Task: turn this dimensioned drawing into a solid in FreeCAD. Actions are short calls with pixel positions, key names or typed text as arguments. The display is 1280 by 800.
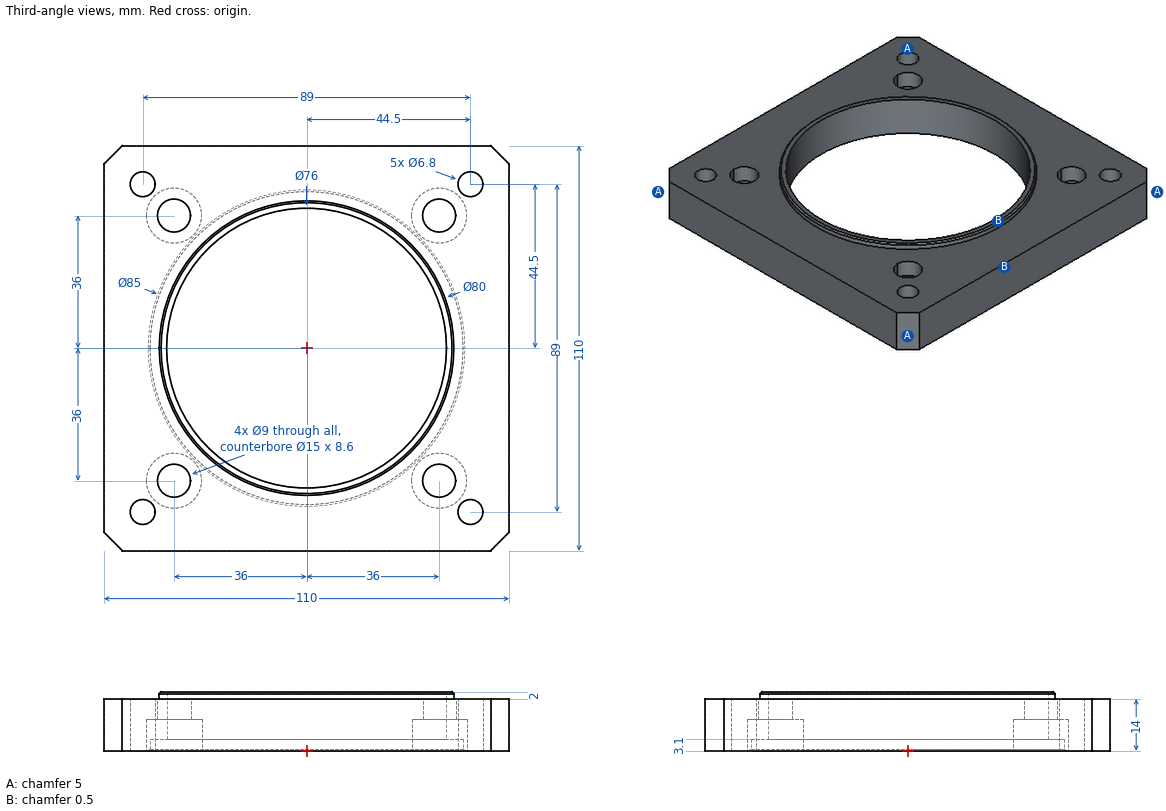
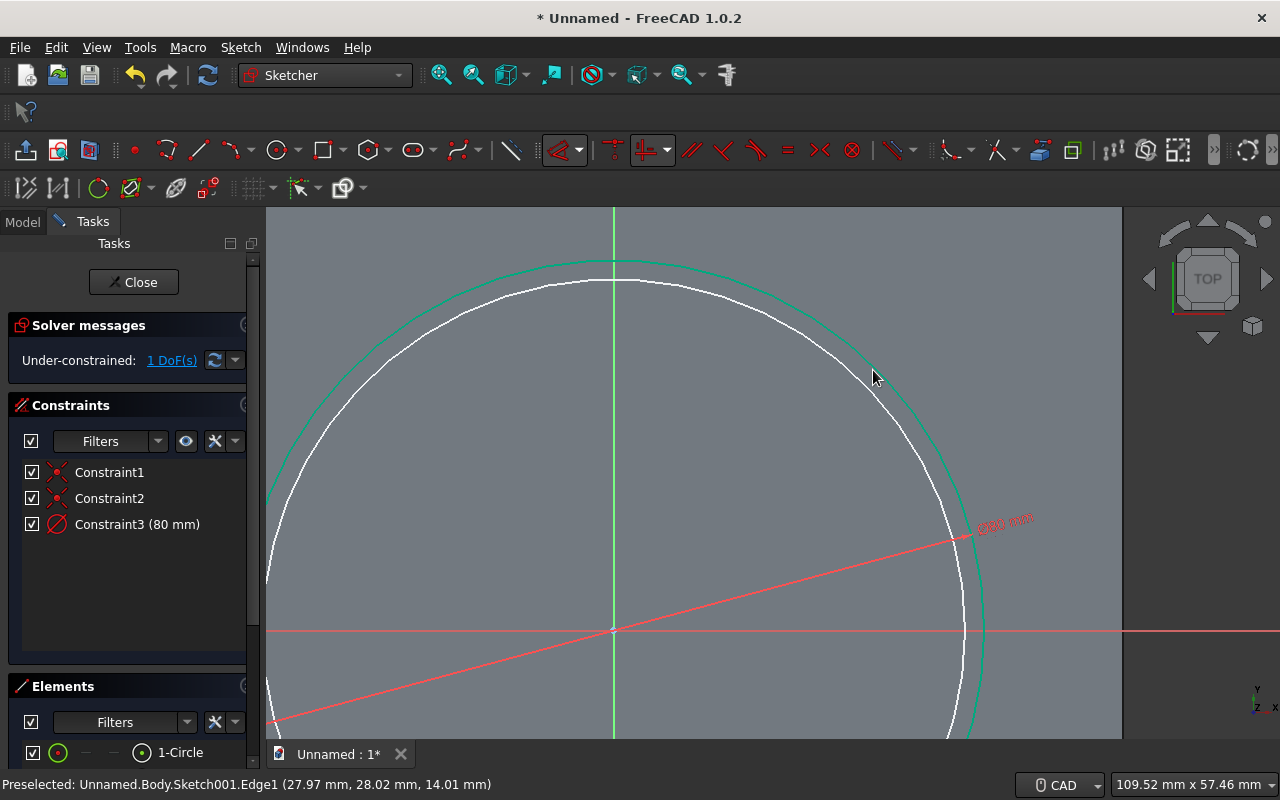
click(861, 381)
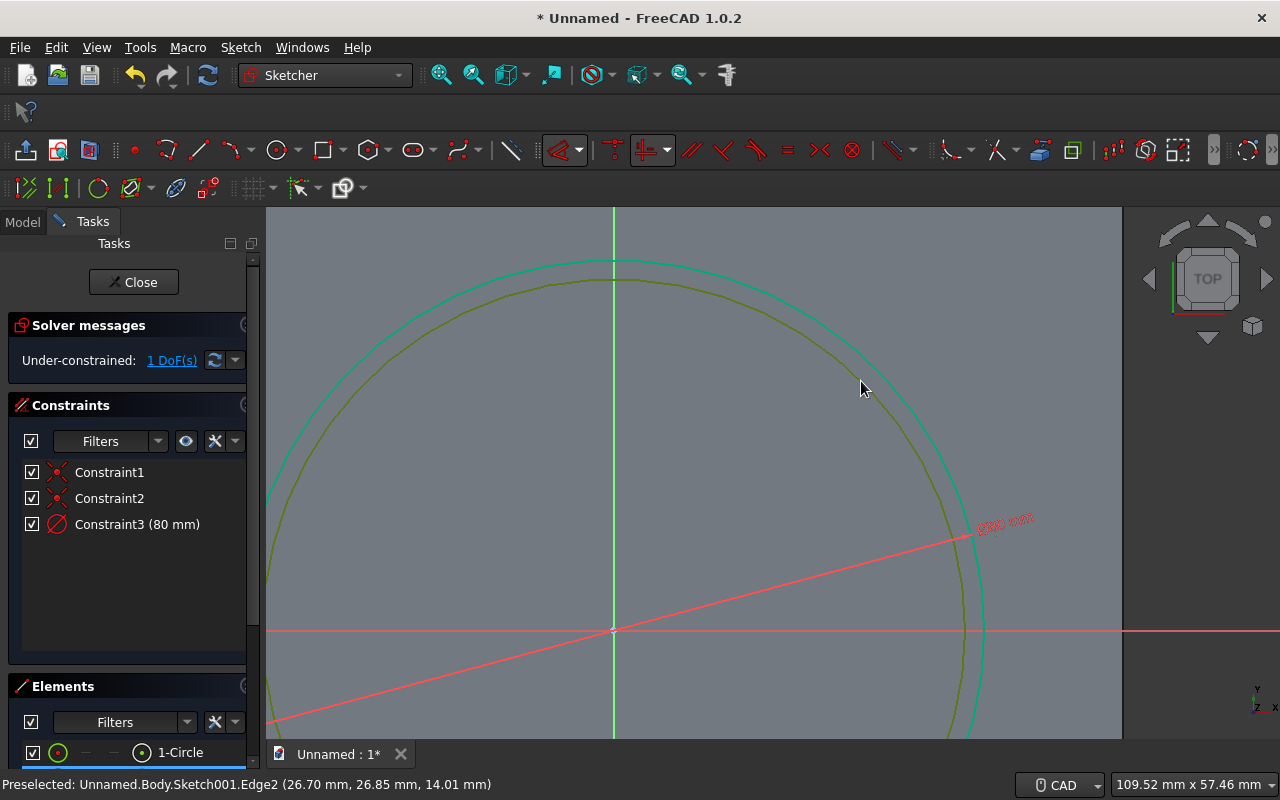
click(582, 150)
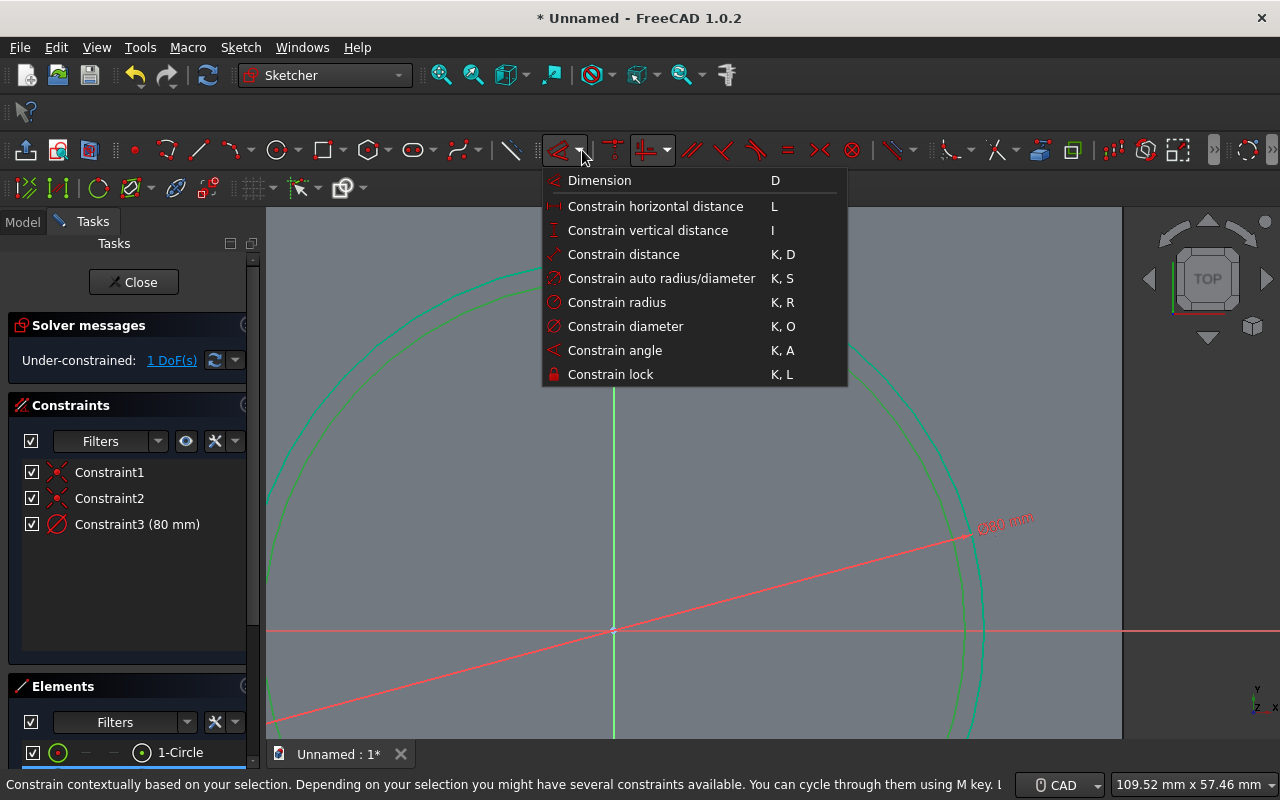
click(695, 326)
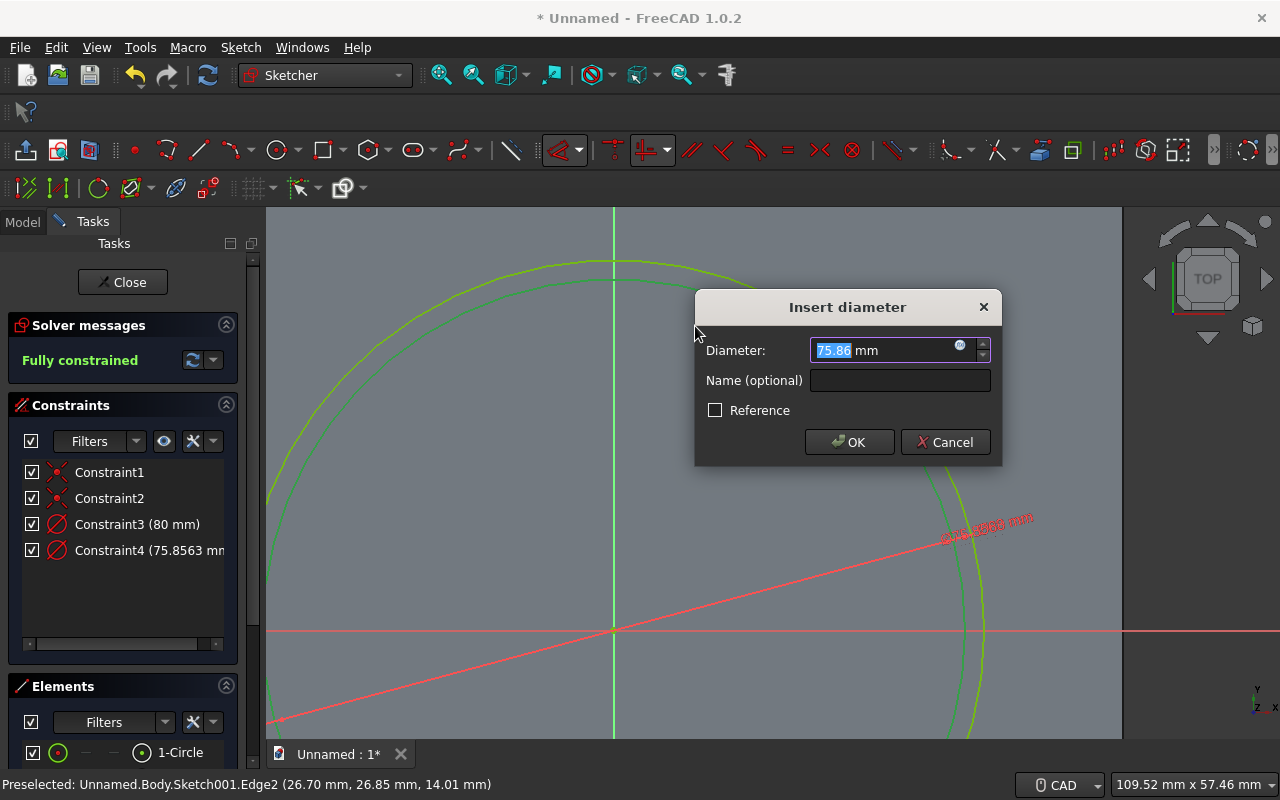
text(76)
key(Return)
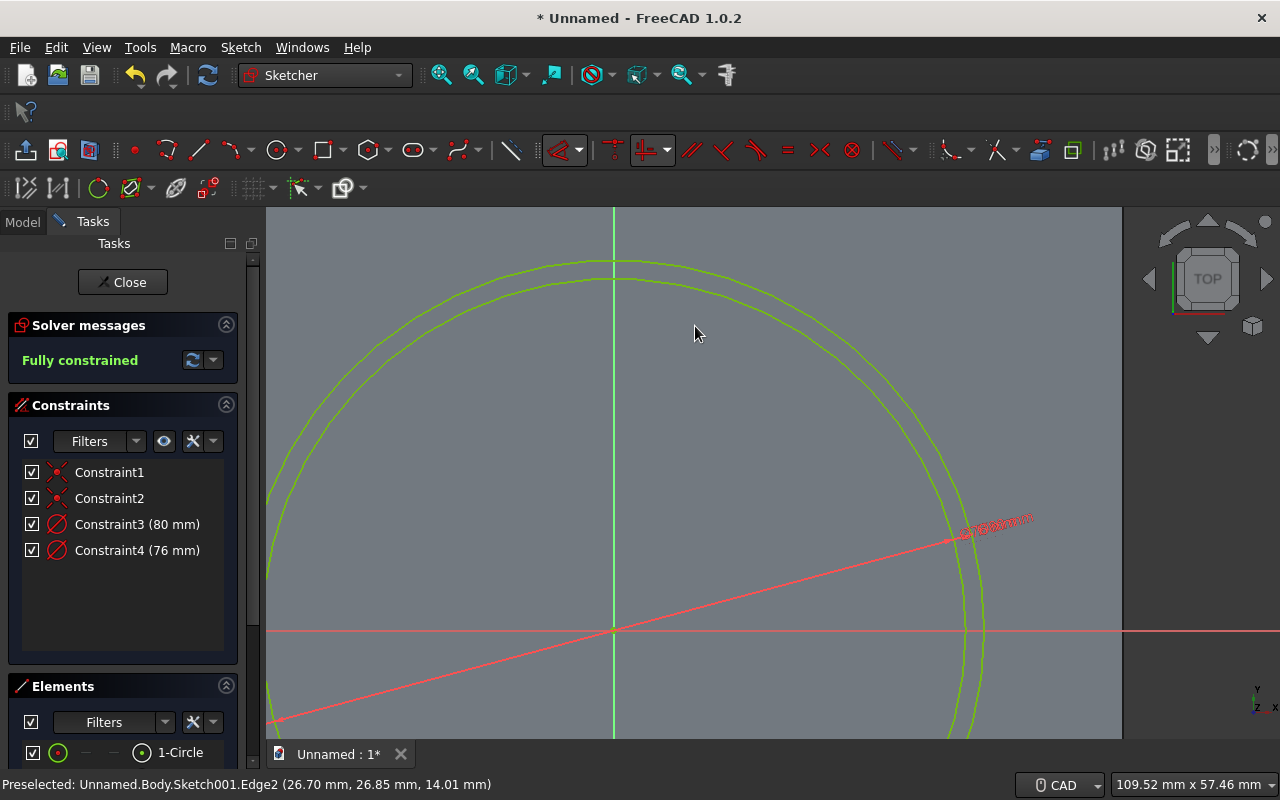
click(123, 282)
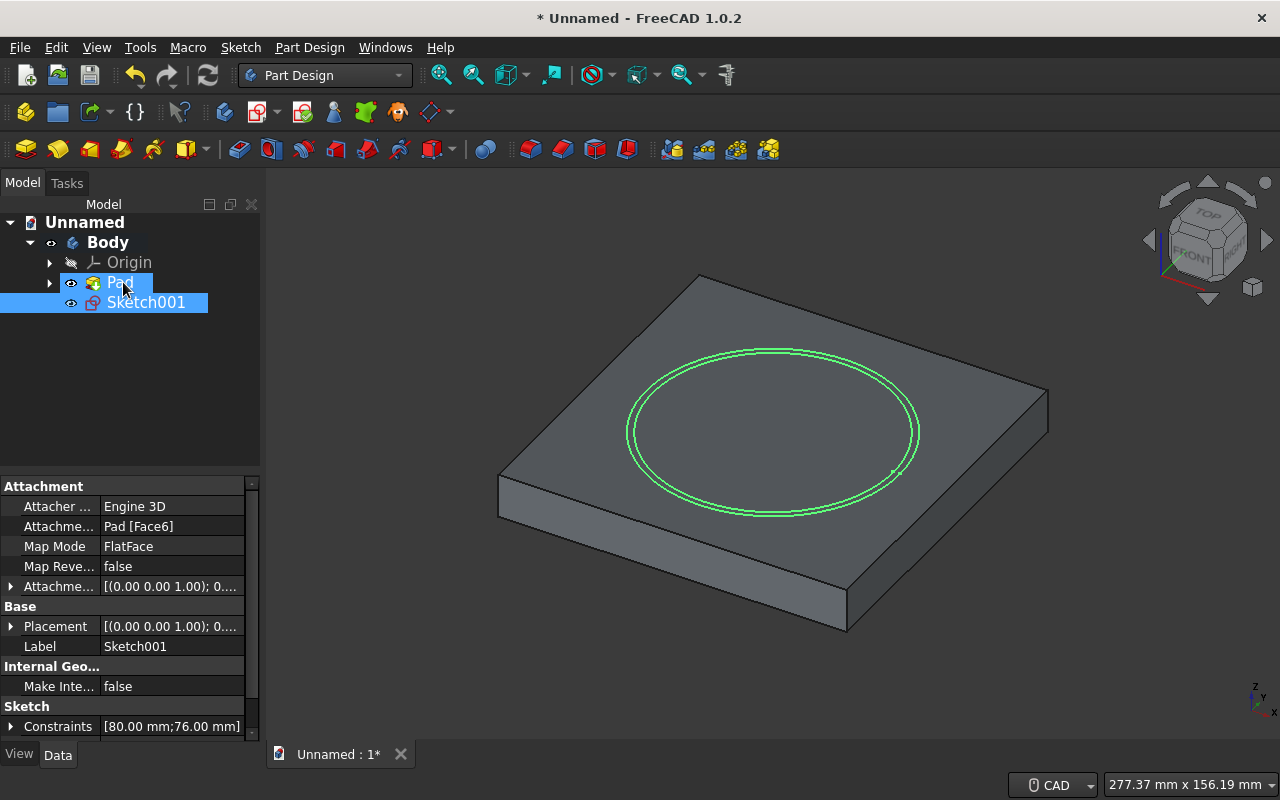
click(26, 150)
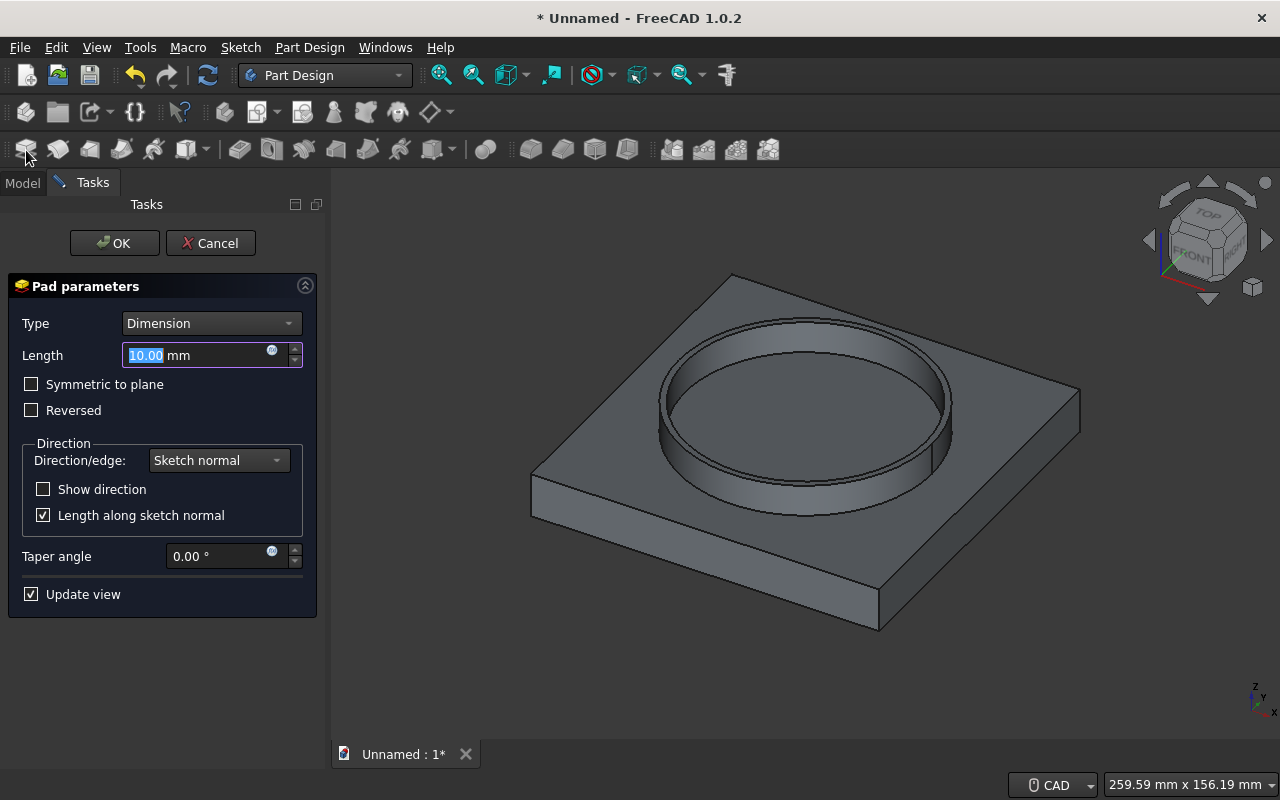
text(2)
key(Tab)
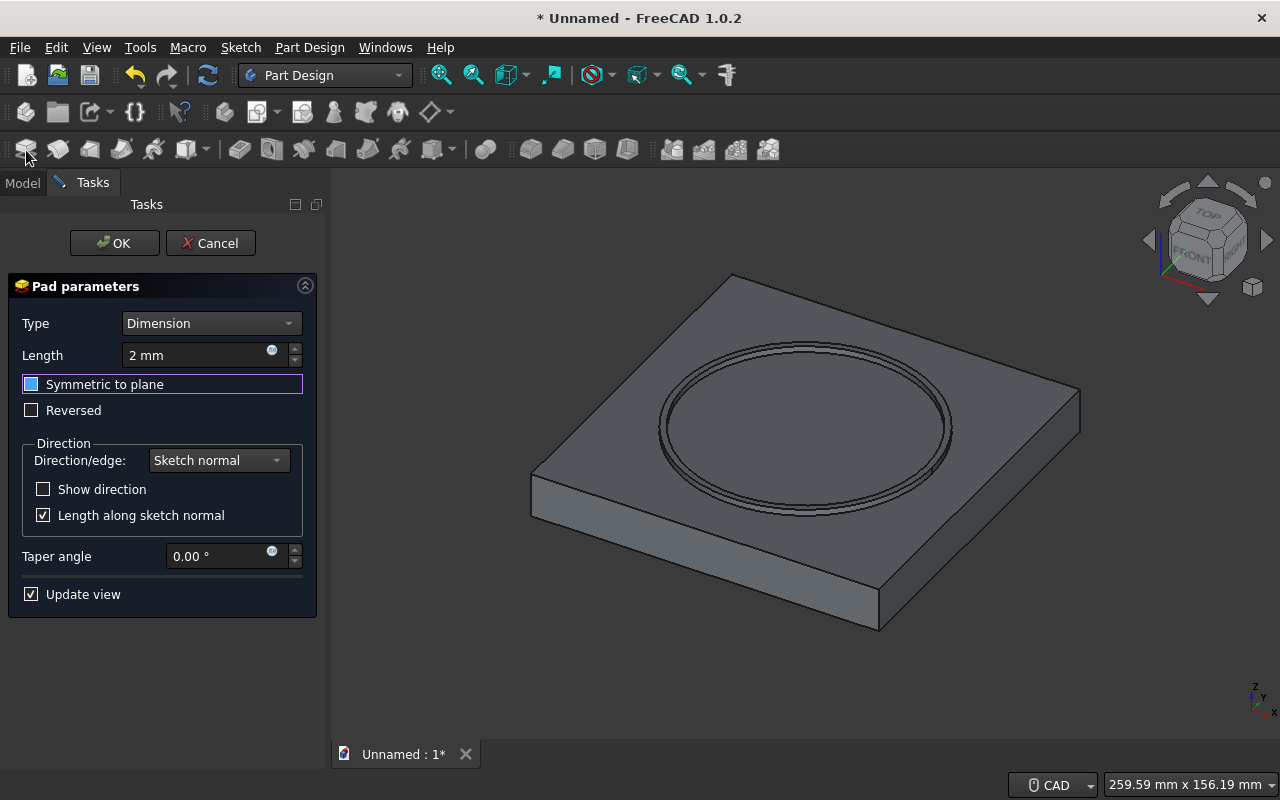
click(115, 243)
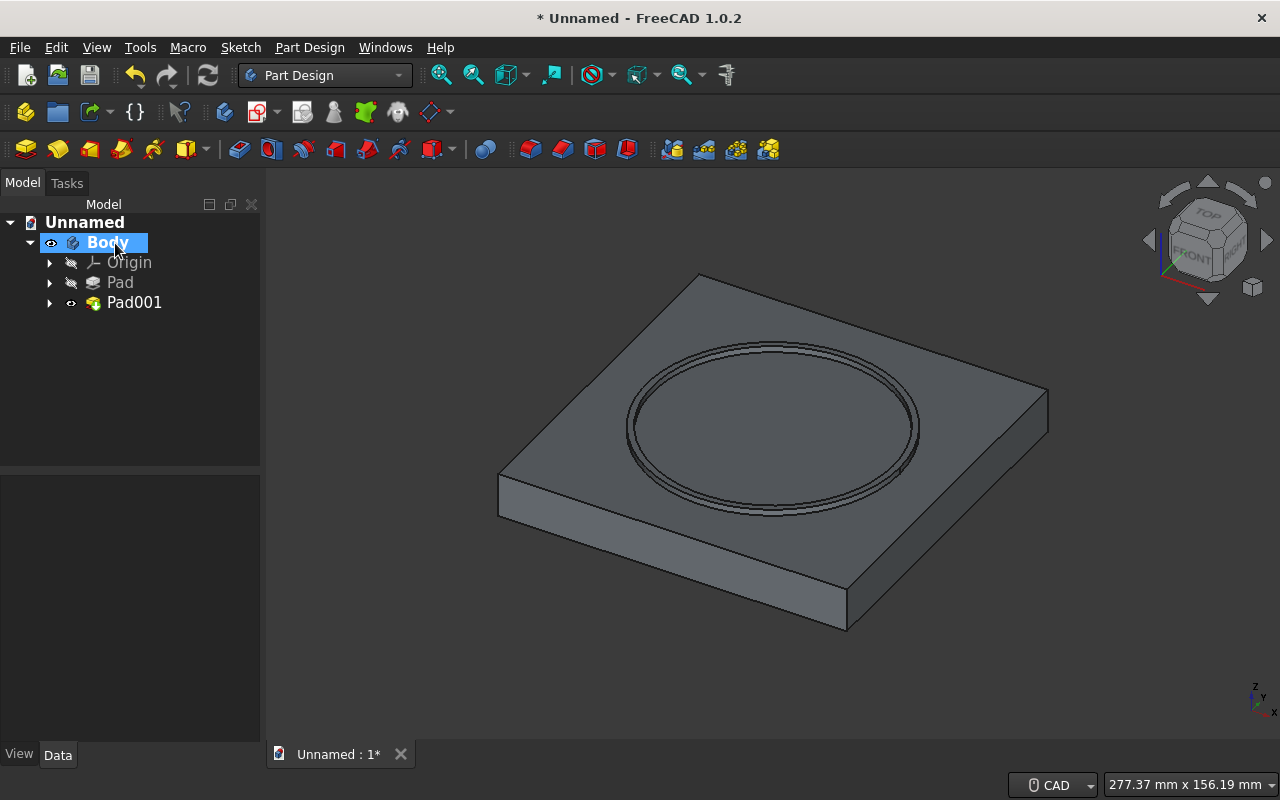
click(1008, 395)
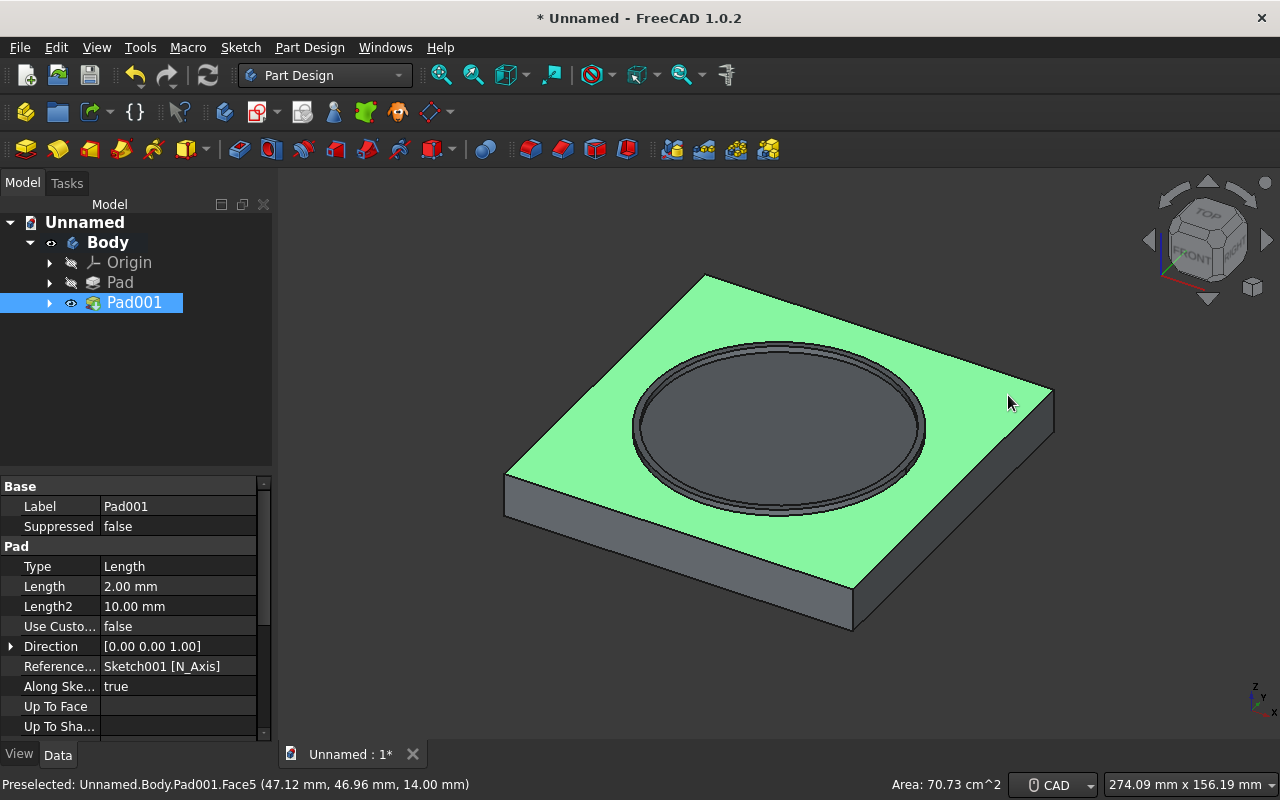
click(258, 112)